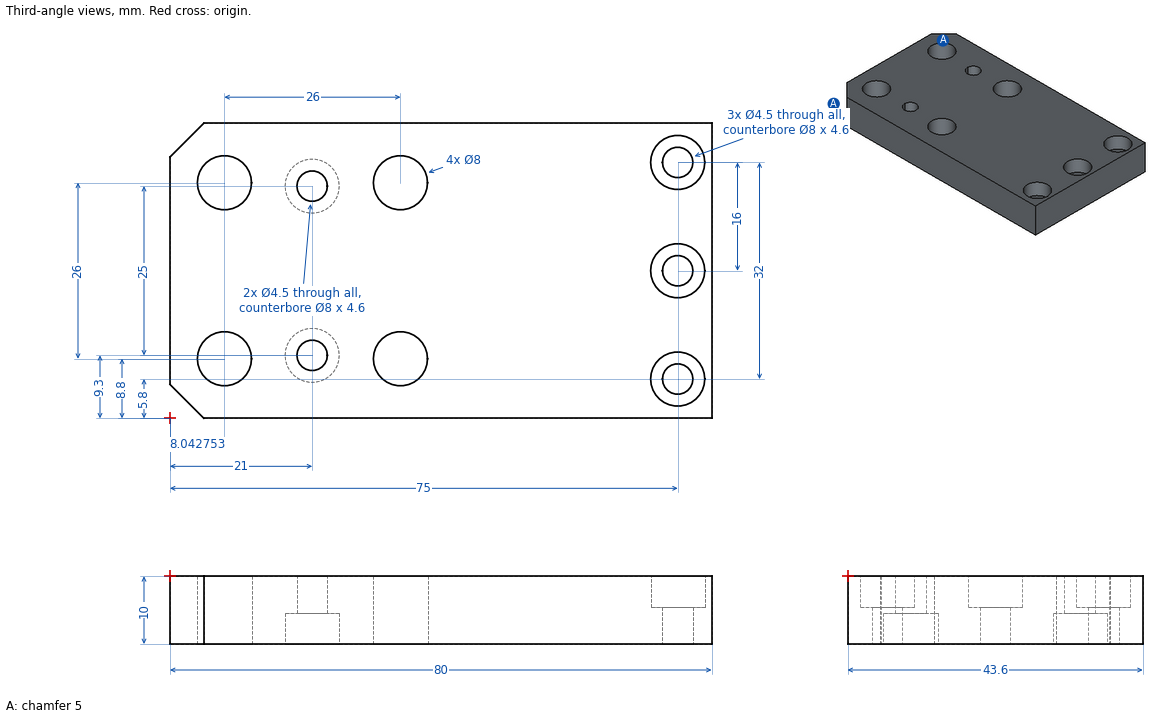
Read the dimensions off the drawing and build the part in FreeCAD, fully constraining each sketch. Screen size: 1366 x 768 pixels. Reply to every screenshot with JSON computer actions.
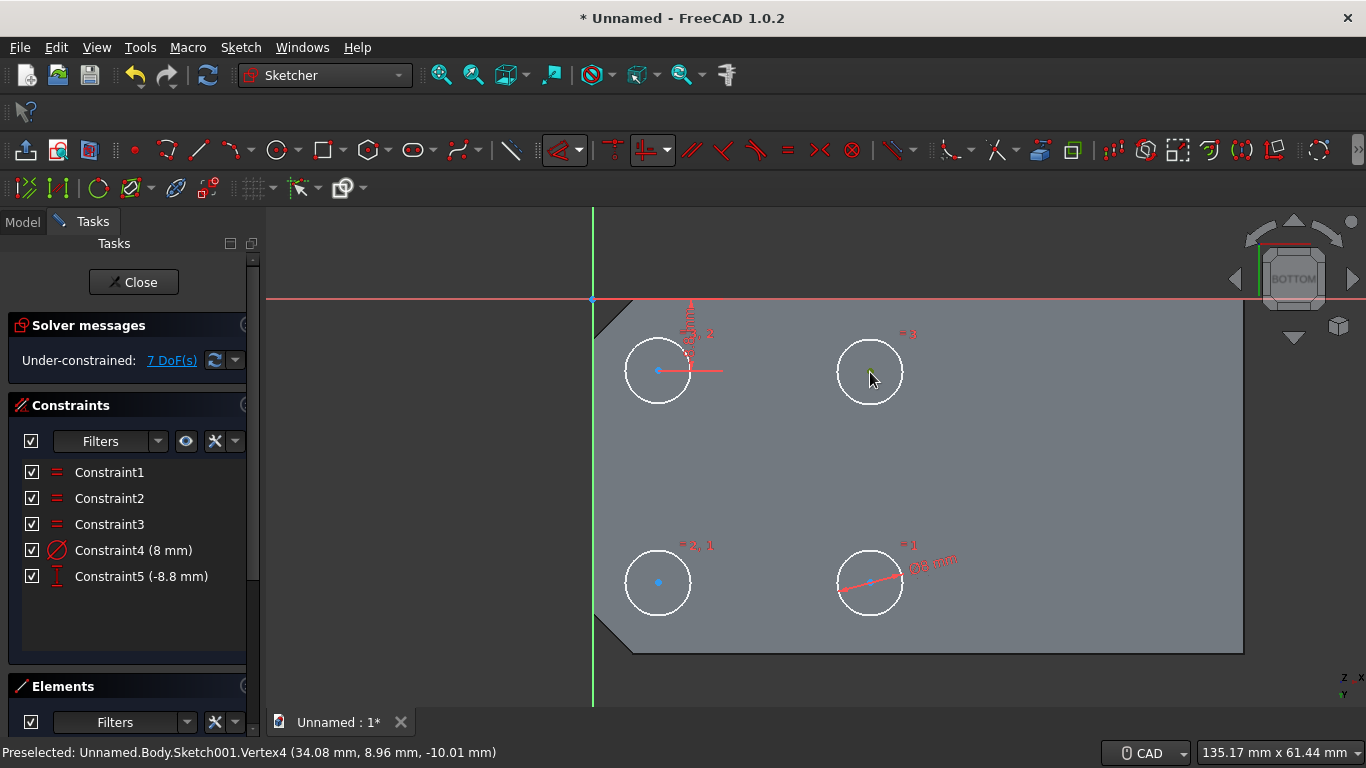
{"action": "left_click", "coordinate": [582, 150]}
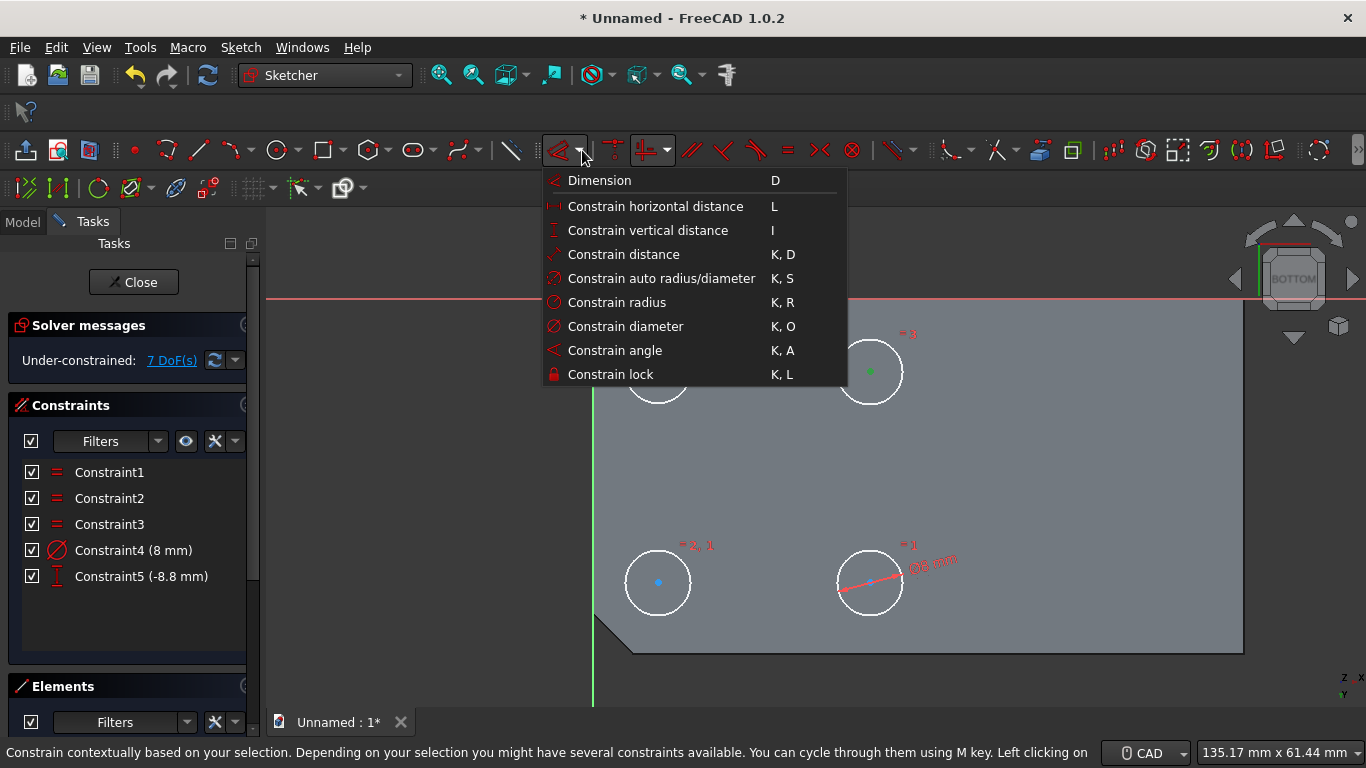
{"action": "left_click", "coordinate": [695, 230]}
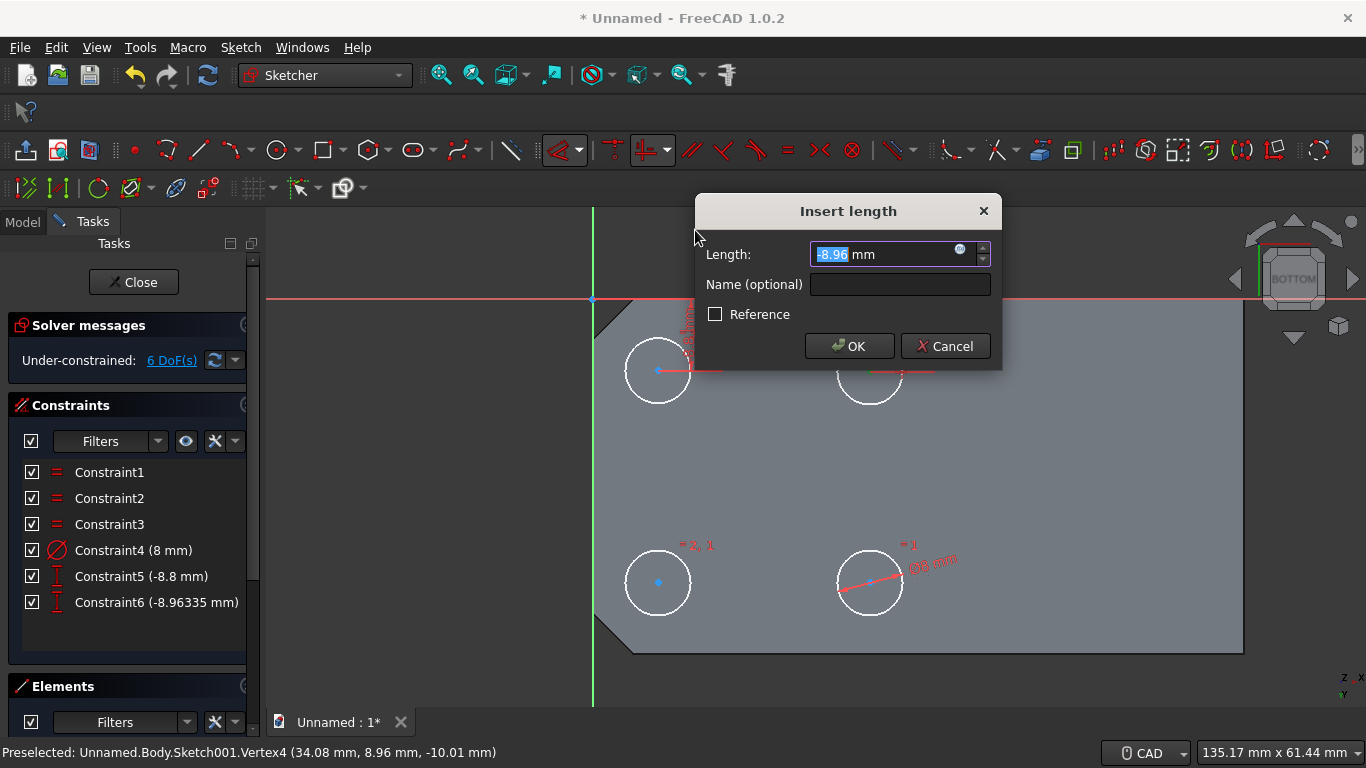
{"action": "type", "text": "-8.8"}
{"action": "key", "text": "Return"}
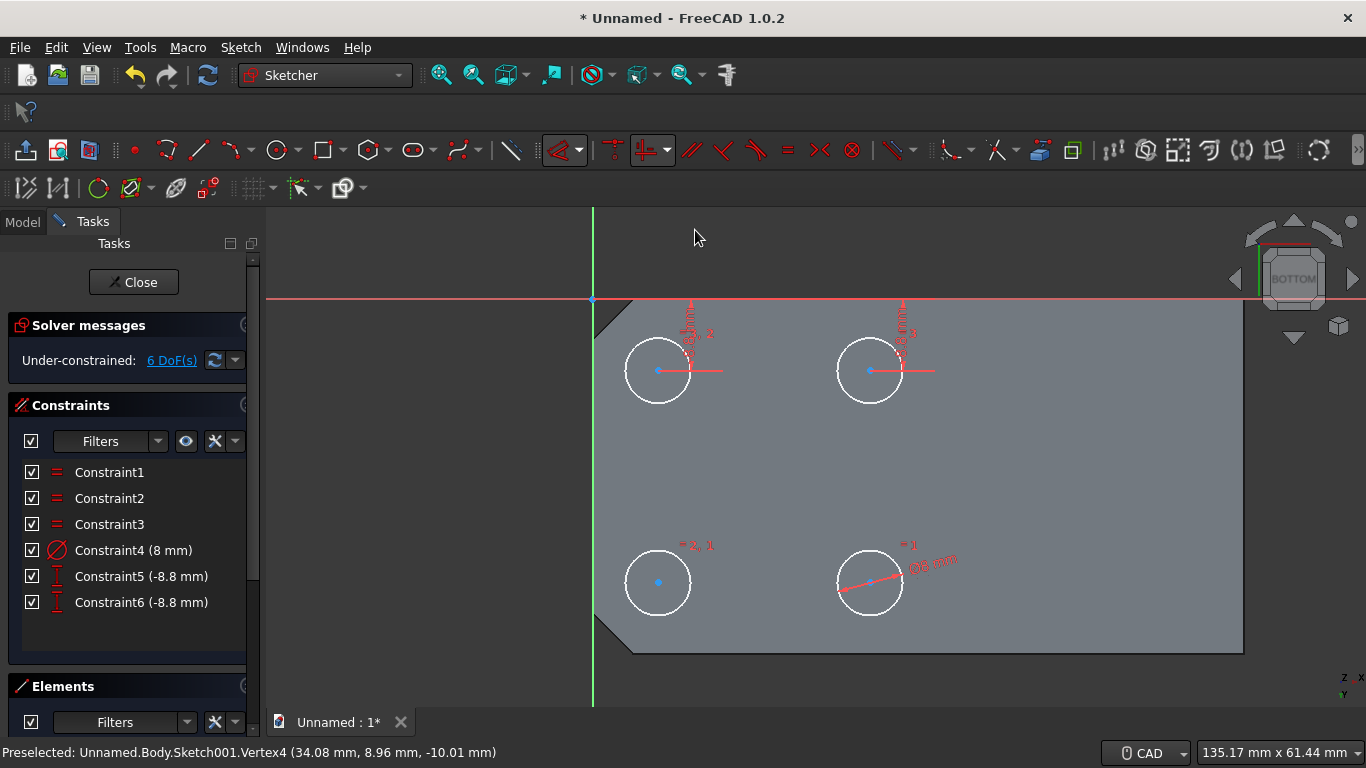
{"action": "left_click", "coordinate": [870, 583]}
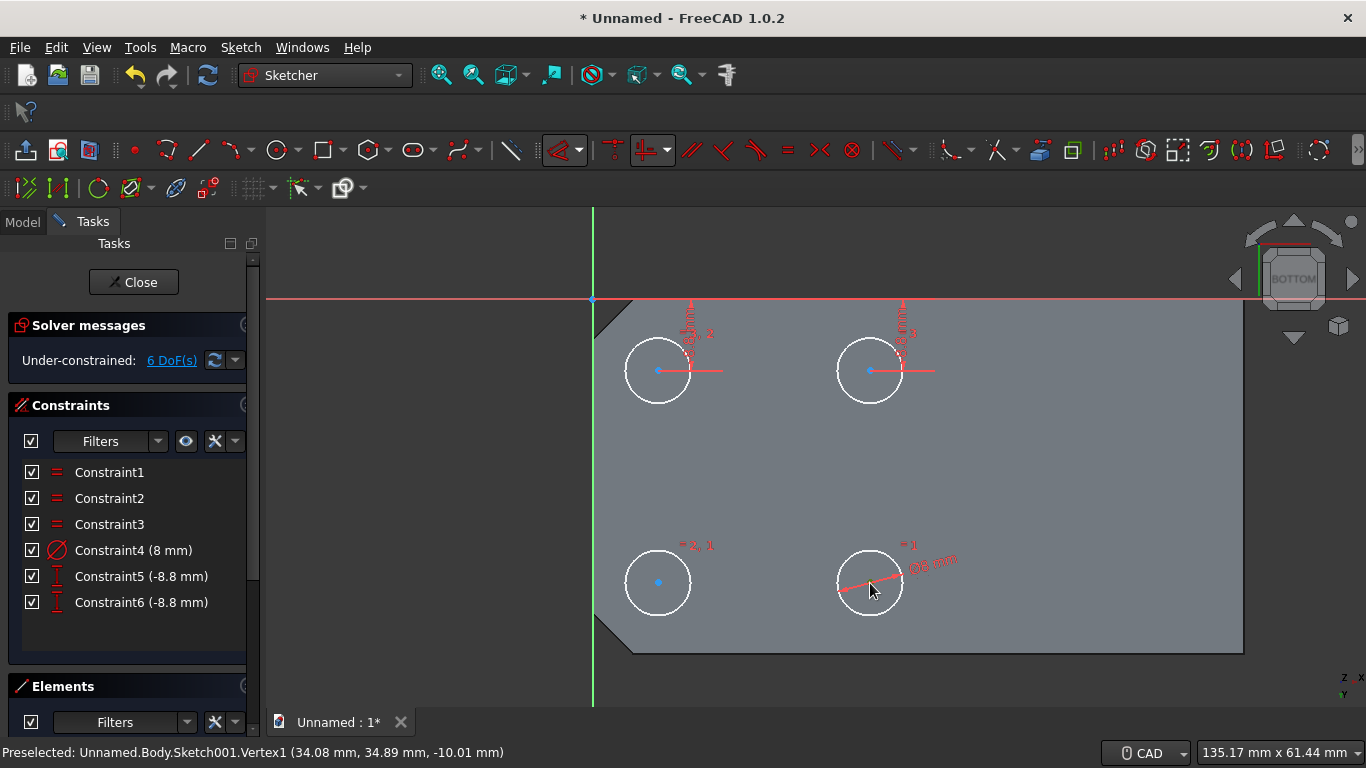
{"action": "left_click", "coordinate": [658, 583]}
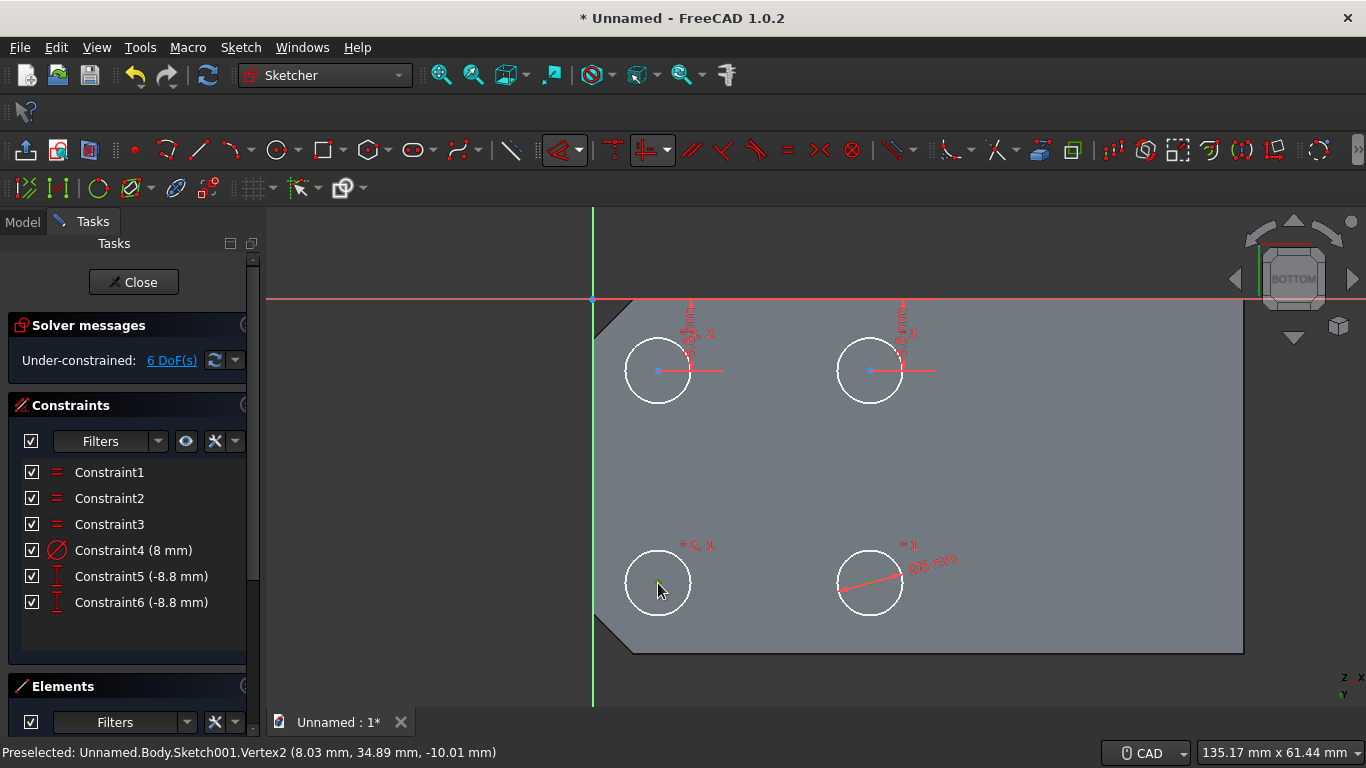
{"action": "left_click", "coordinate": [582, 150]}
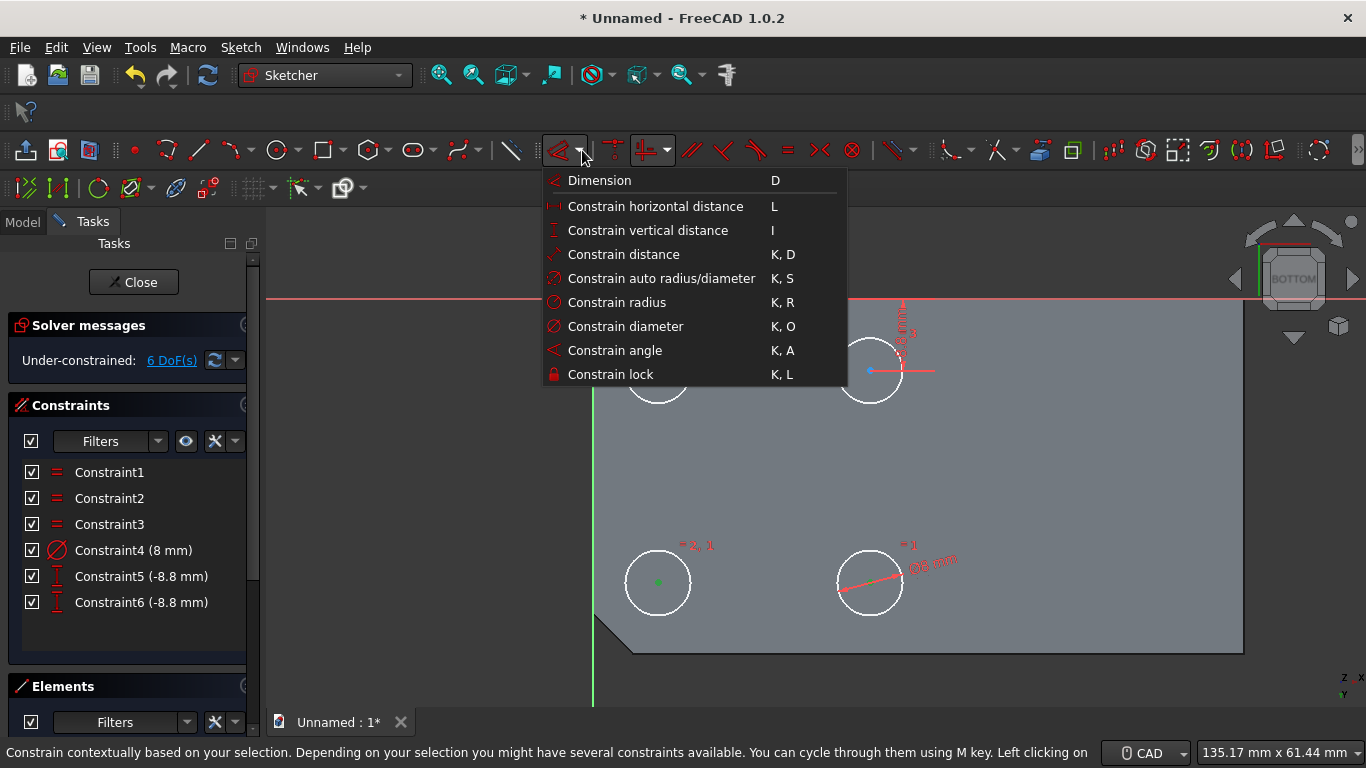
{"action": "left_click", "coordinate": [695, 206]}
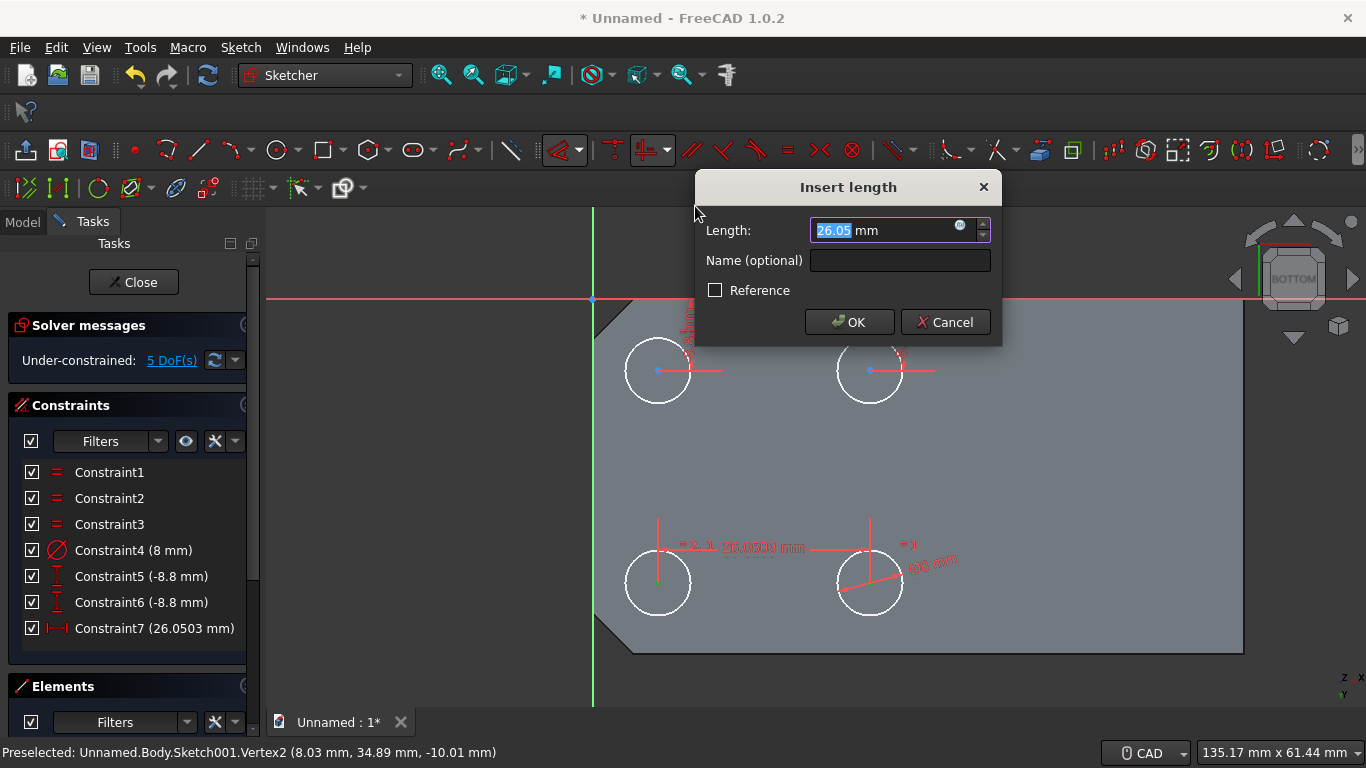
{"action": "type", "text": "26"}
{"action": "key", "text": "Return"}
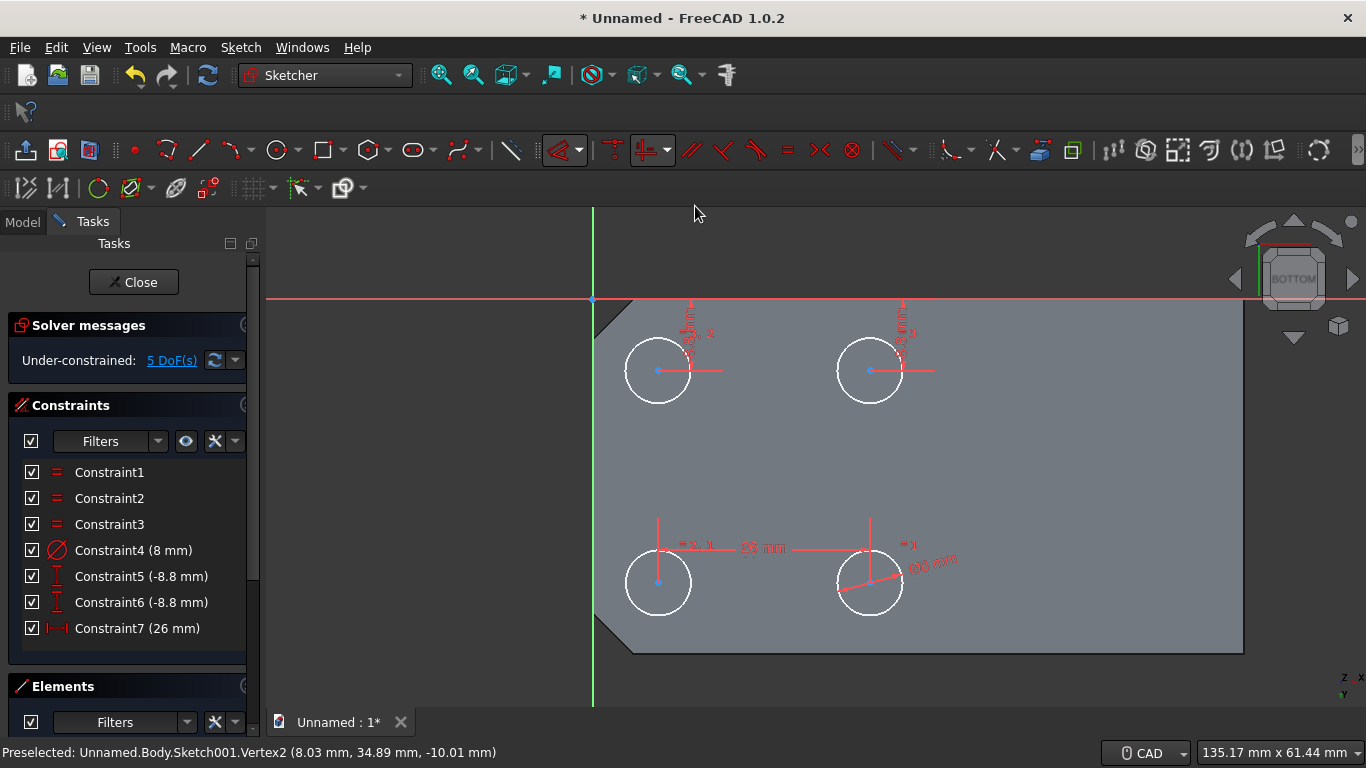
{"action": "left_click", "coordinate": [870, 583]}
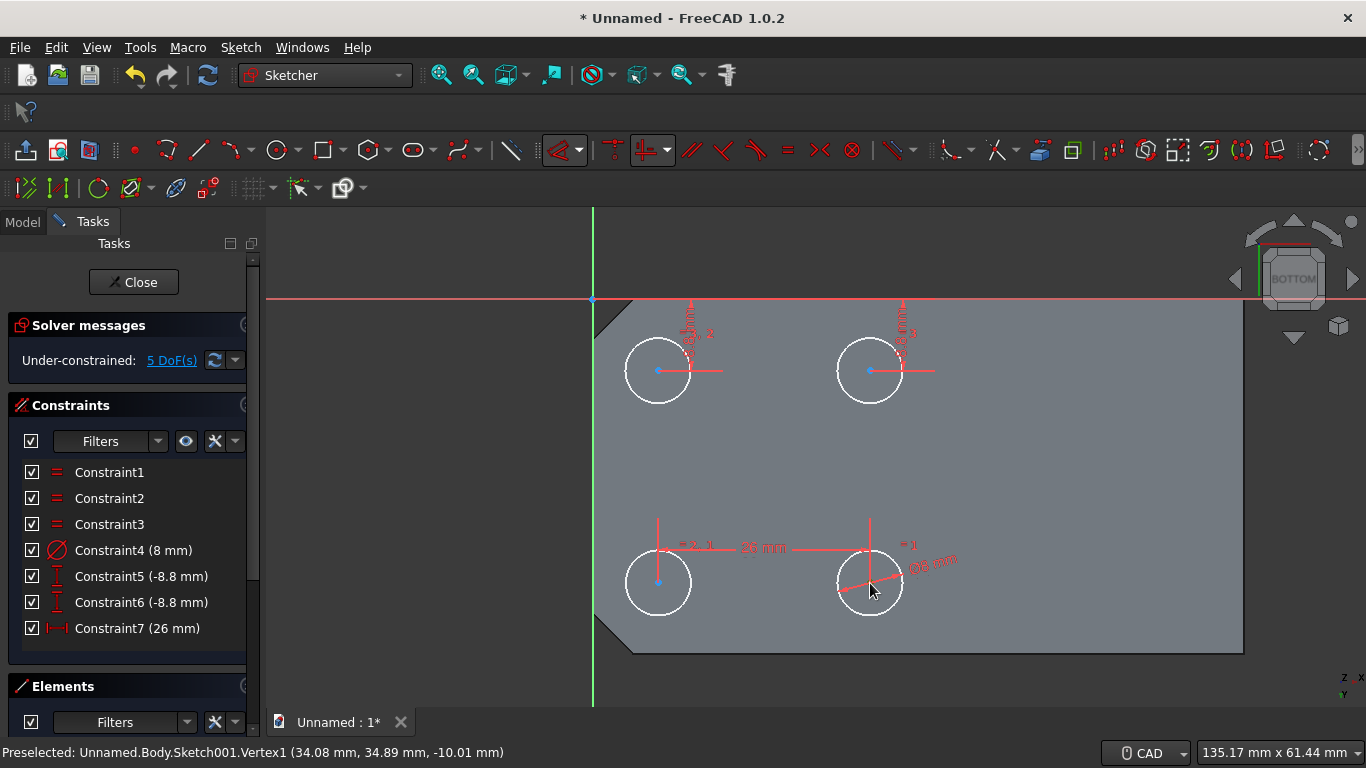
{"action": "left_click", "coordinate": [658, 371]}